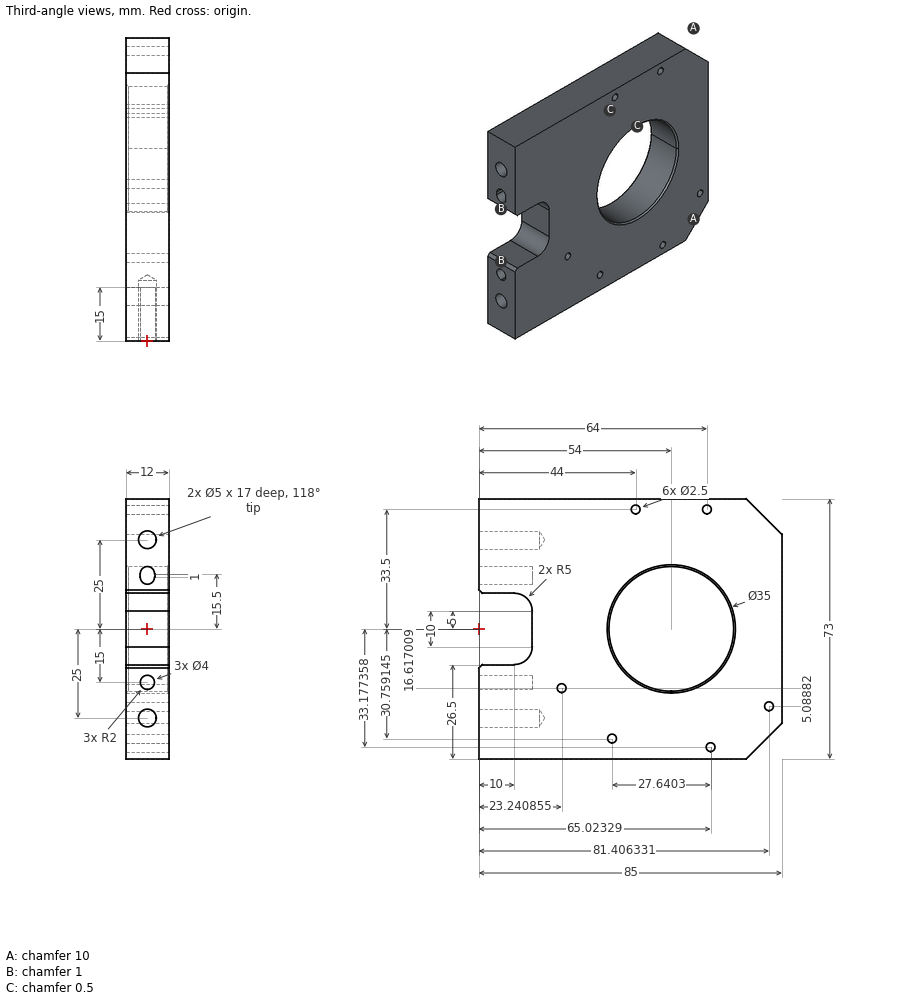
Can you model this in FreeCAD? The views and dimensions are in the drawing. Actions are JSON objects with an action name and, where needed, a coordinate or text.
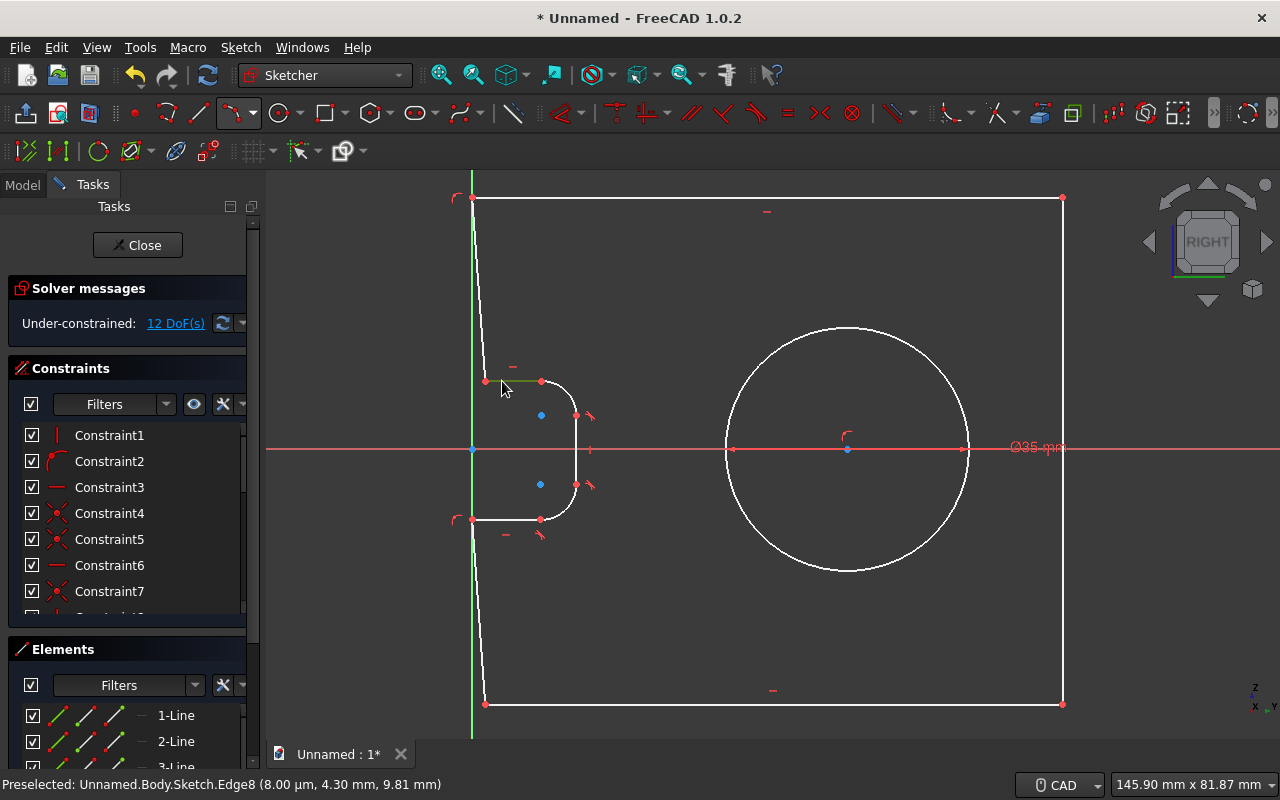
{"action": "left_click", "coordinate": [573, 400]}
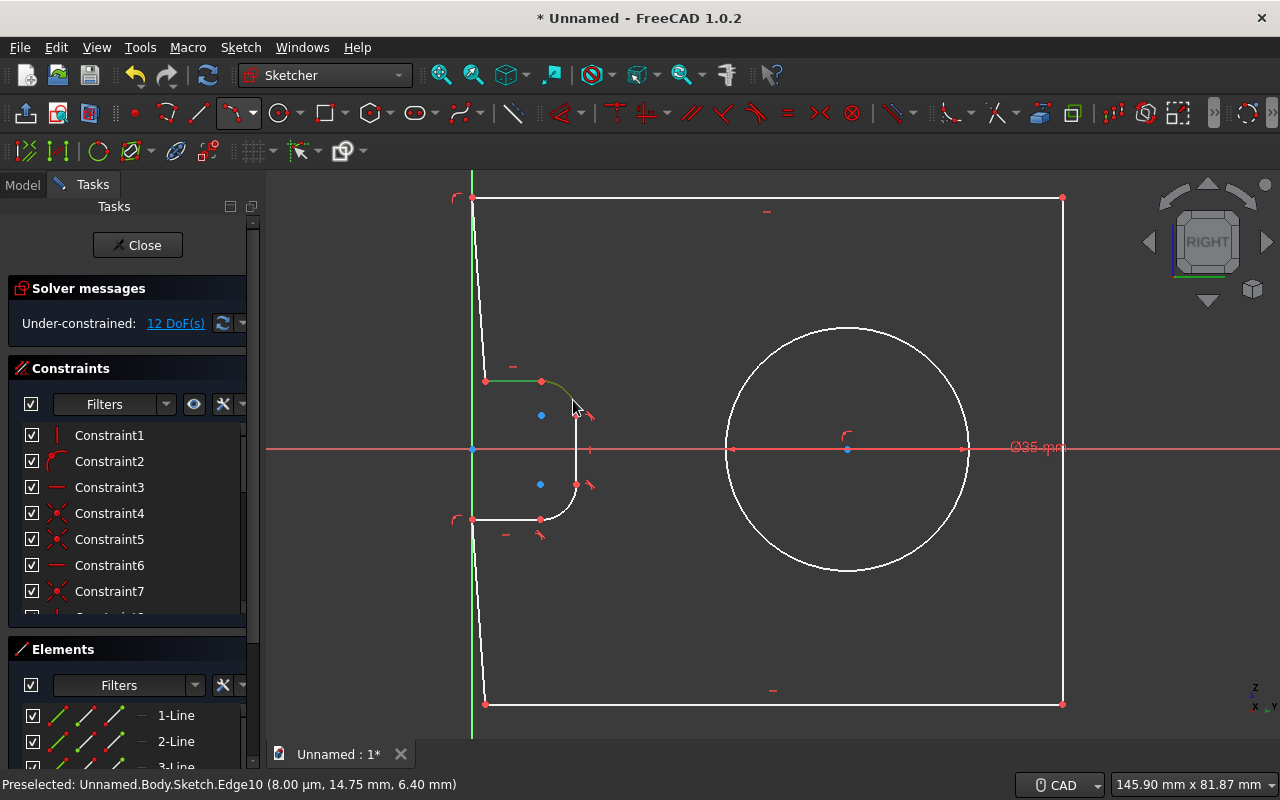
{"action": "left_click", "coordinate": [756, 114]}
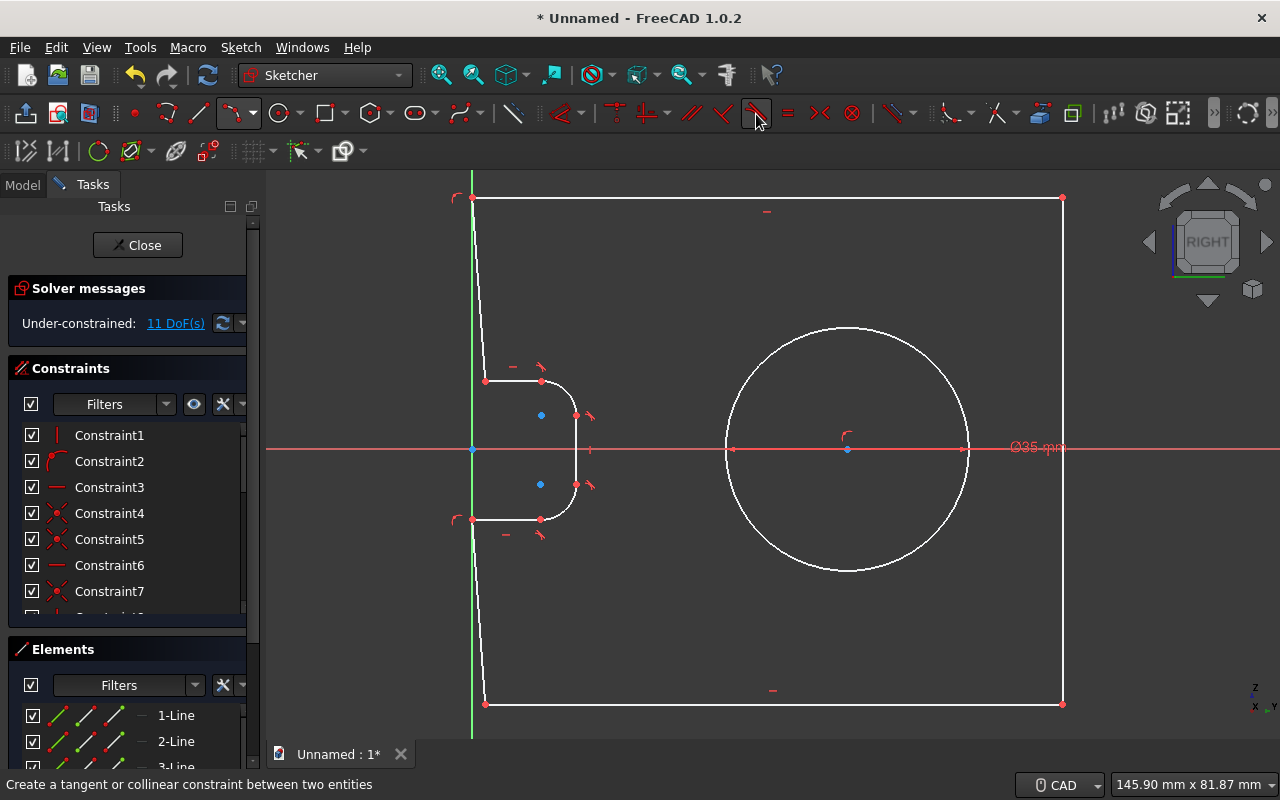
{"action": "left_click", "coordinate": [476, 575]}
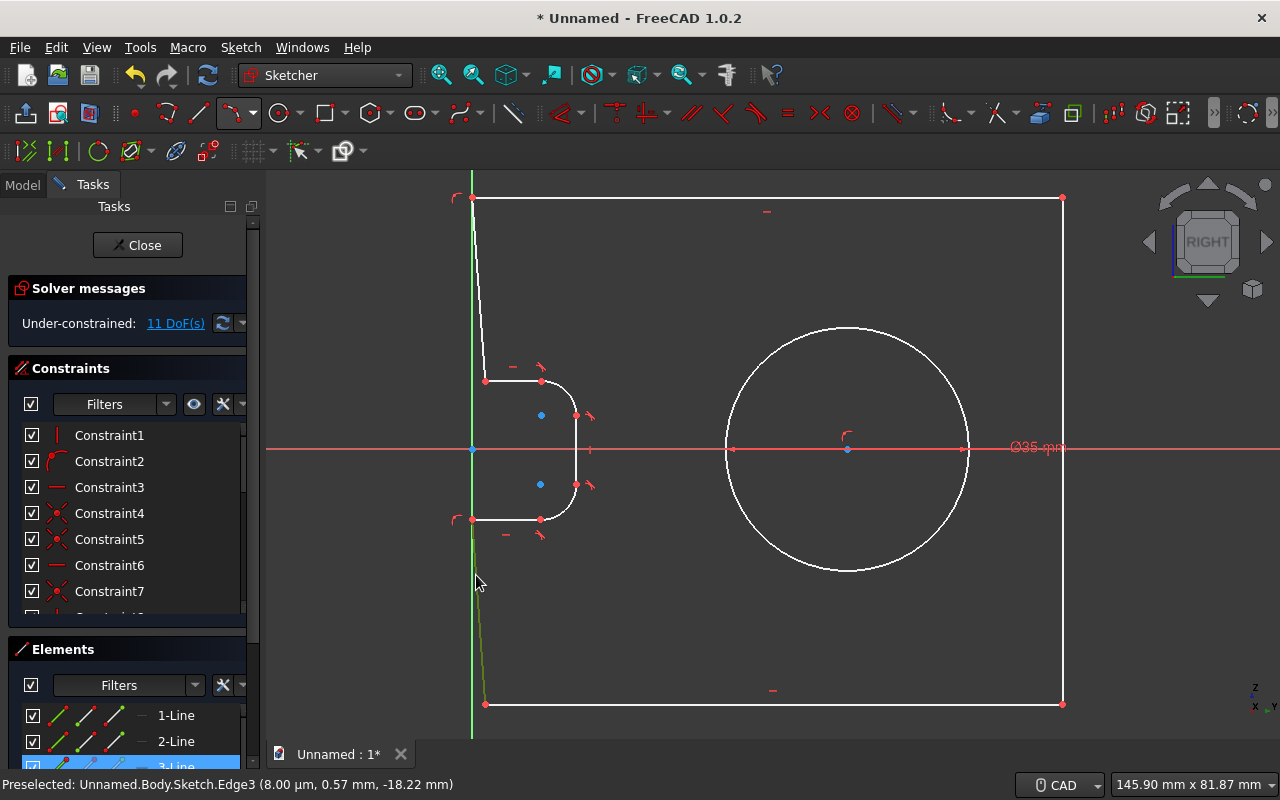
{"action": "left_click", "coordinate": [670, 114]}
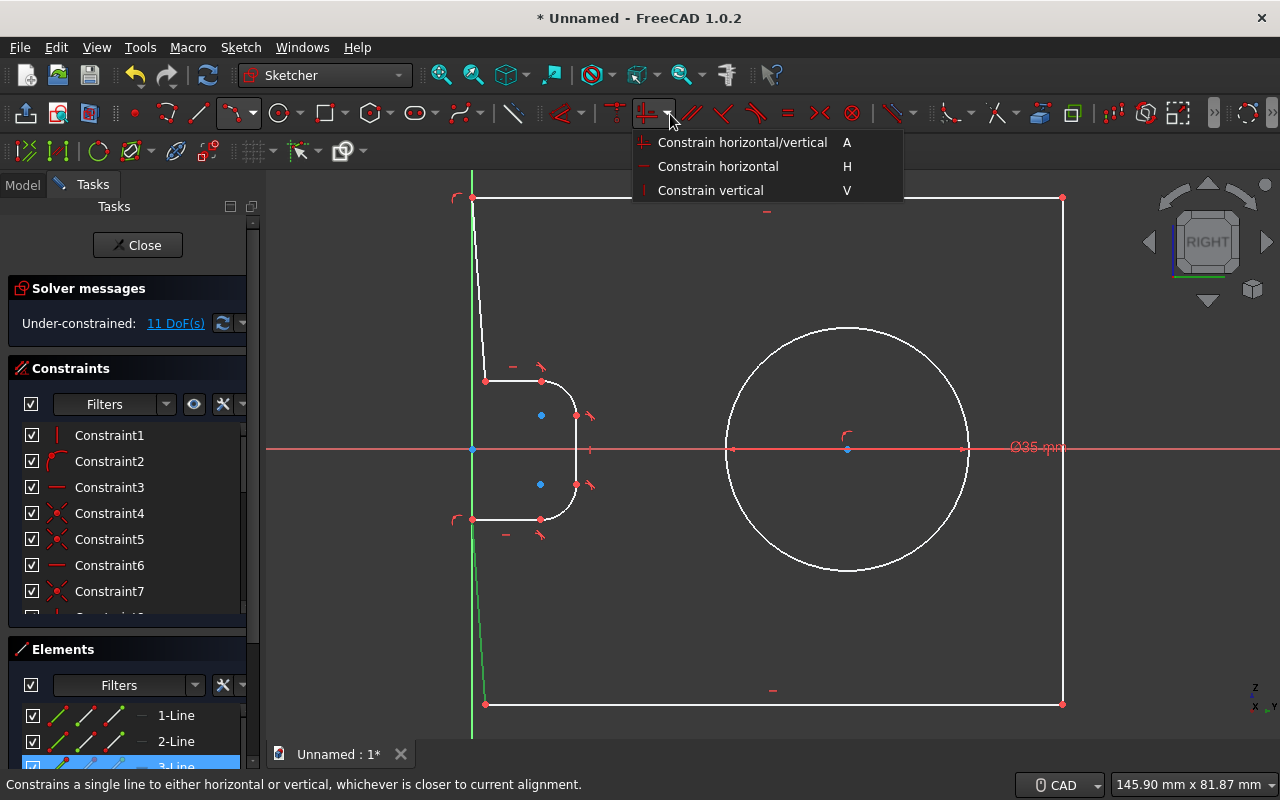
{"action": "left_click", "coordinate": [768, 190]}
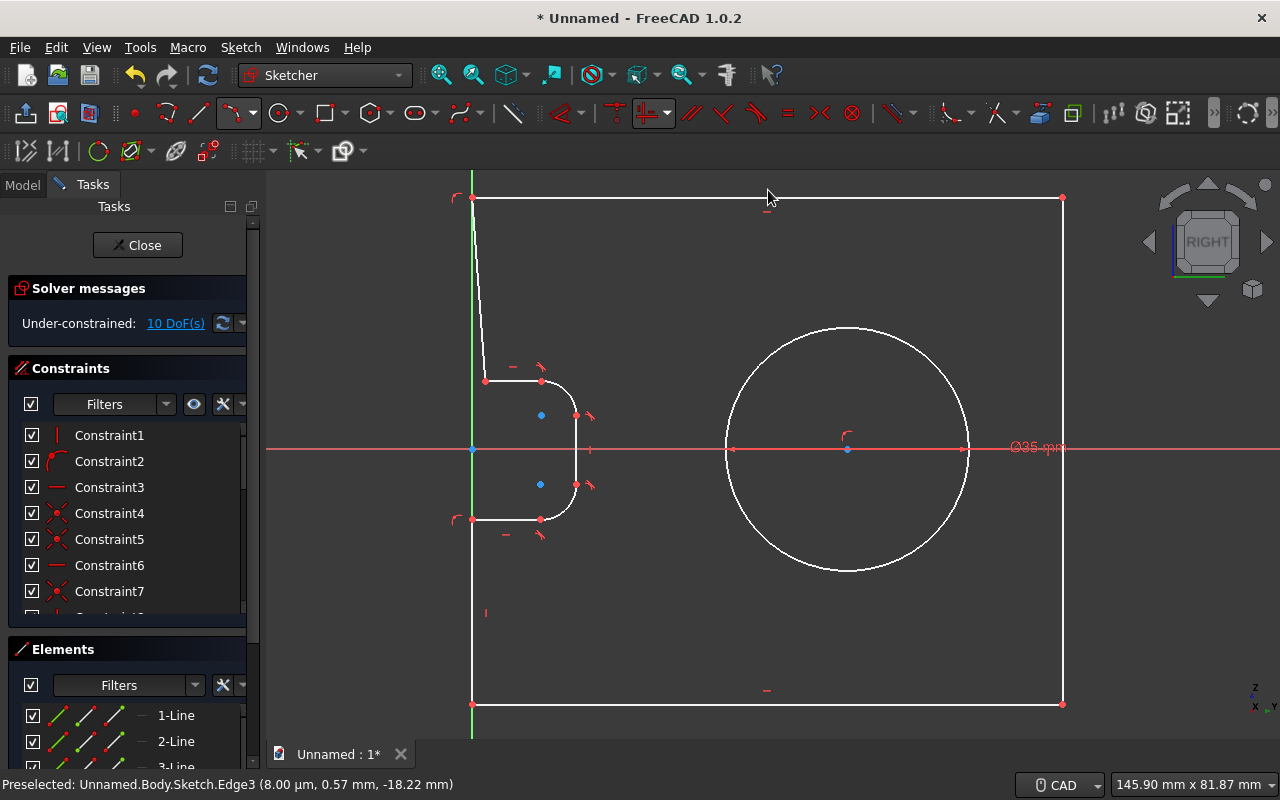
{"action": "left_click", "coordinate": [476, 253]}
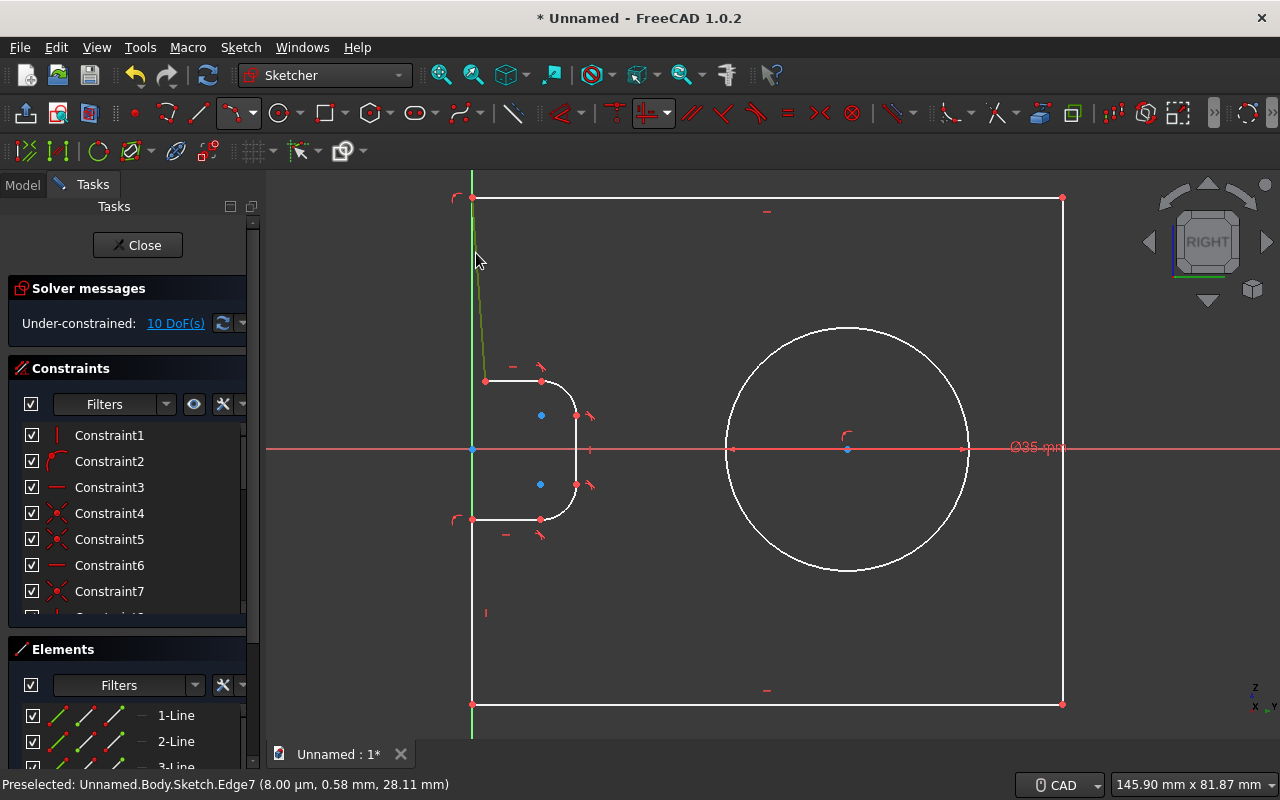
{"action": "left_click", "coordinate": [670, 114]}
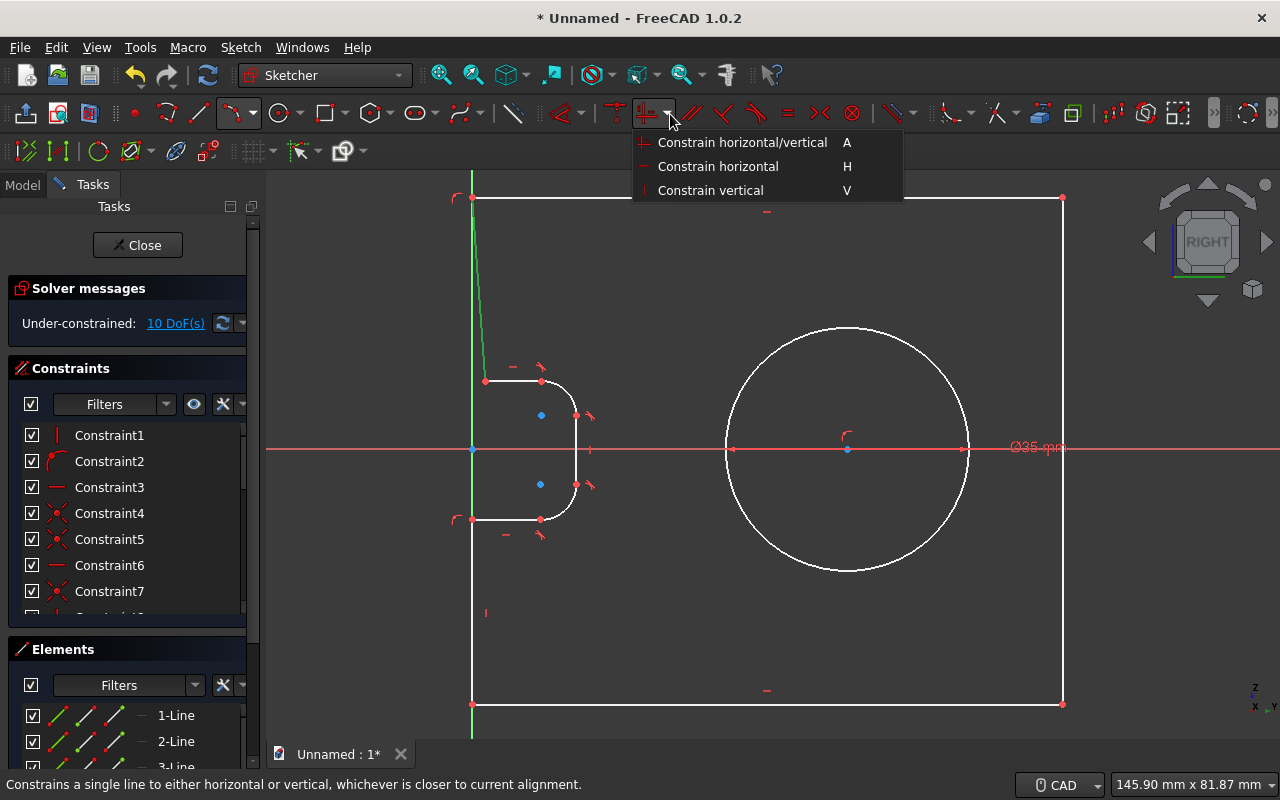
{"action": "left_click", "coordinate": [768, 190]}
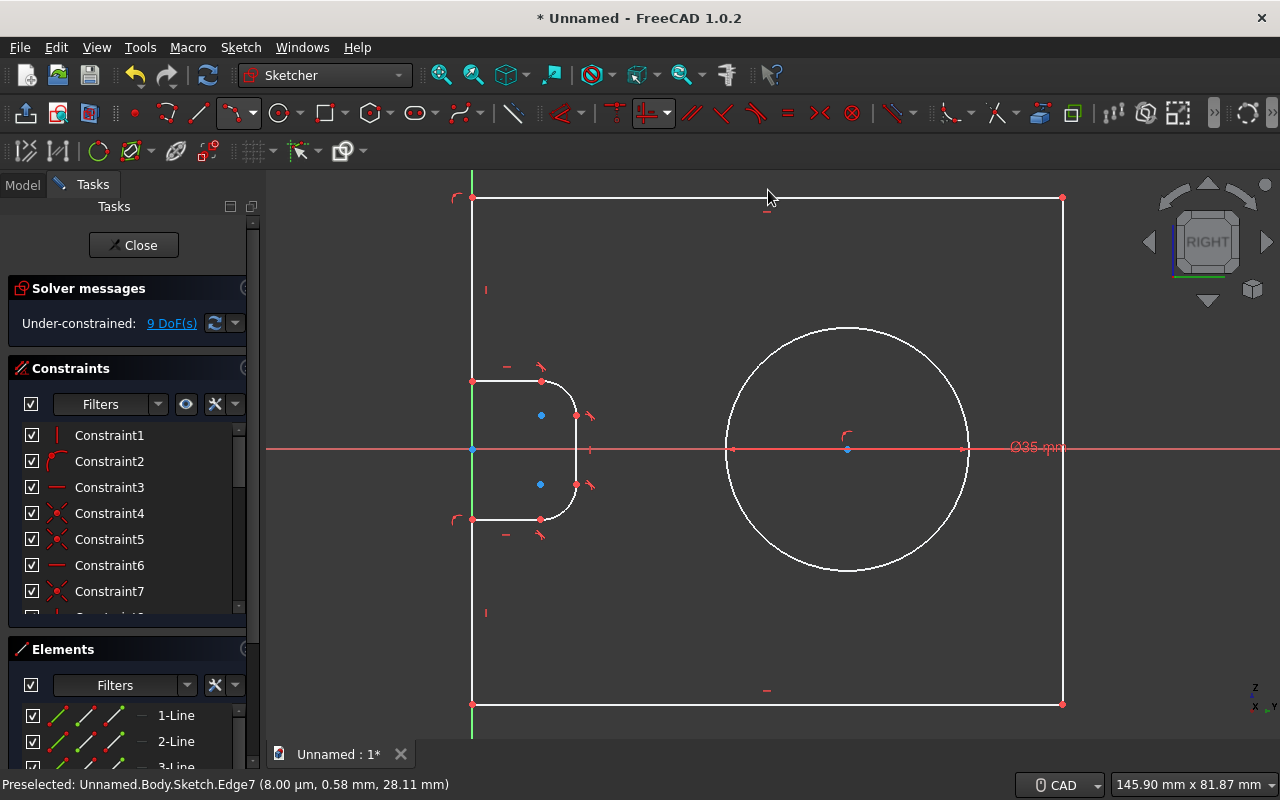
{"action": "left_click", "coordinate": [557, 516]}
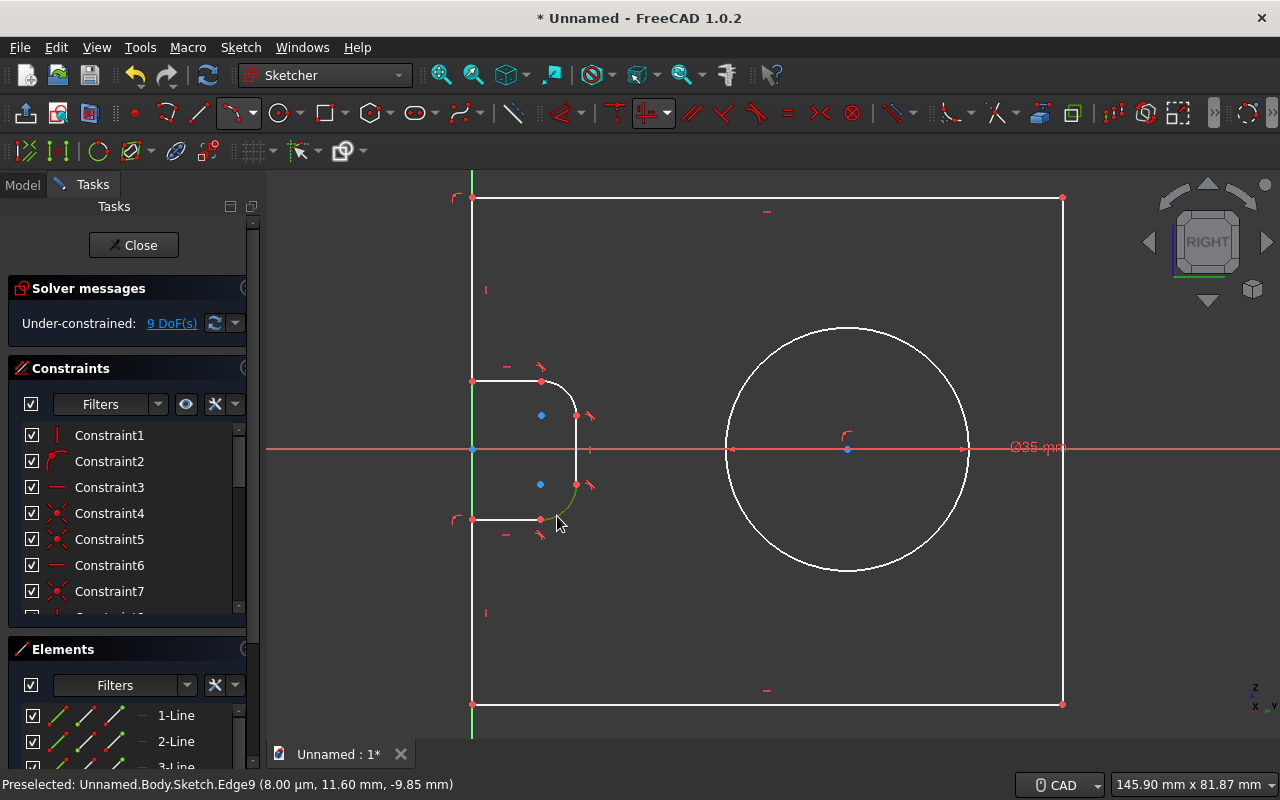
{"action": "left_click", "coordinate": [573, 400]}